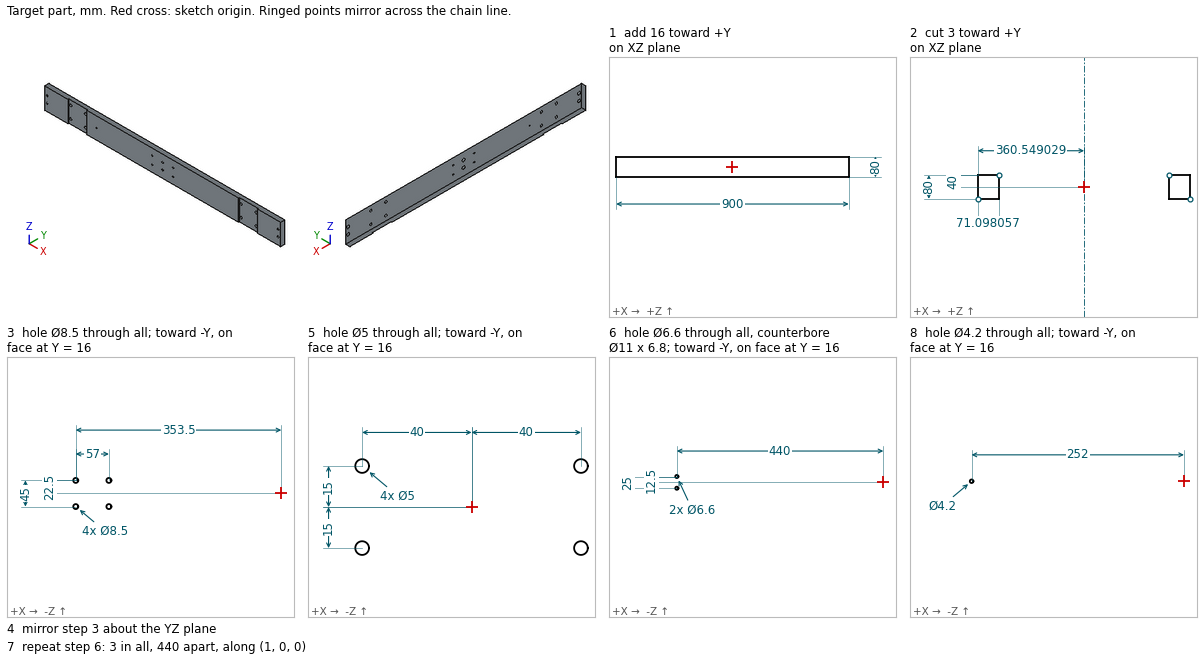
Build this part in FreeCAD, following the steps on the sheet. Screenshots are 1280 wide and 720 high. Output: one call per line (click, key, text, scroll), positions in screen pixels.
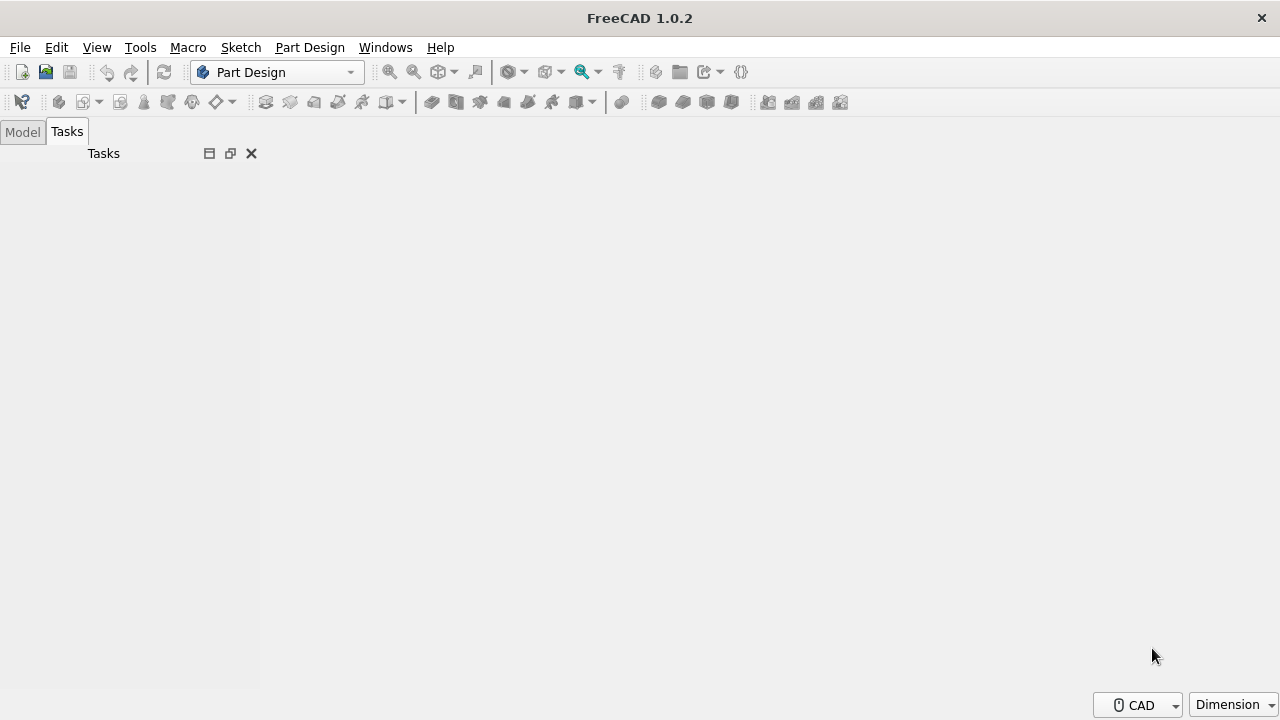
click(22, 72)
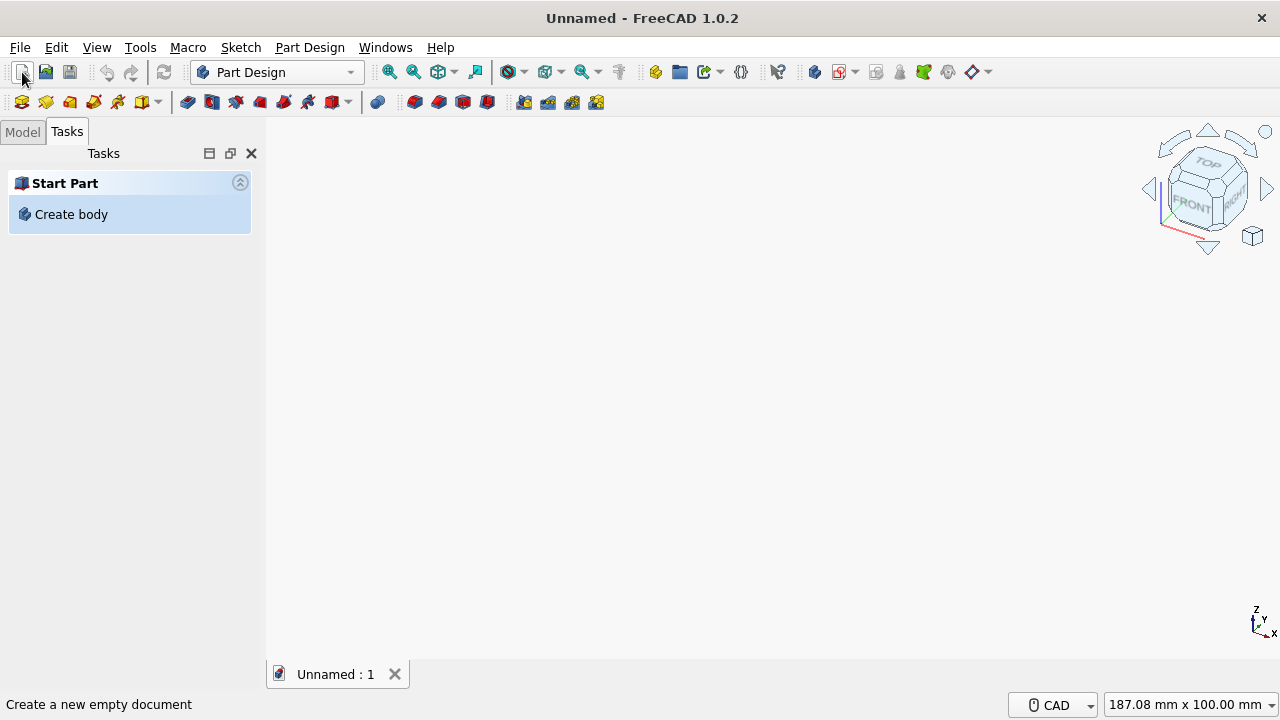
click(840, 72)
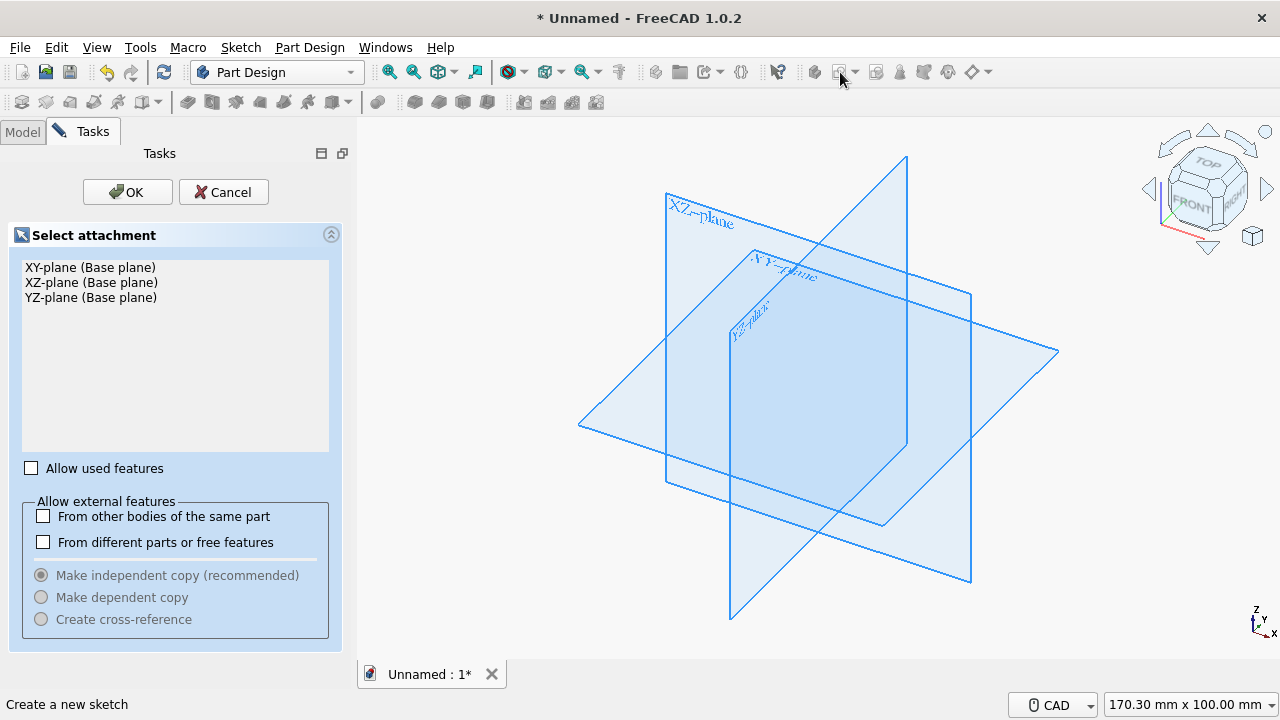
click(82, 282)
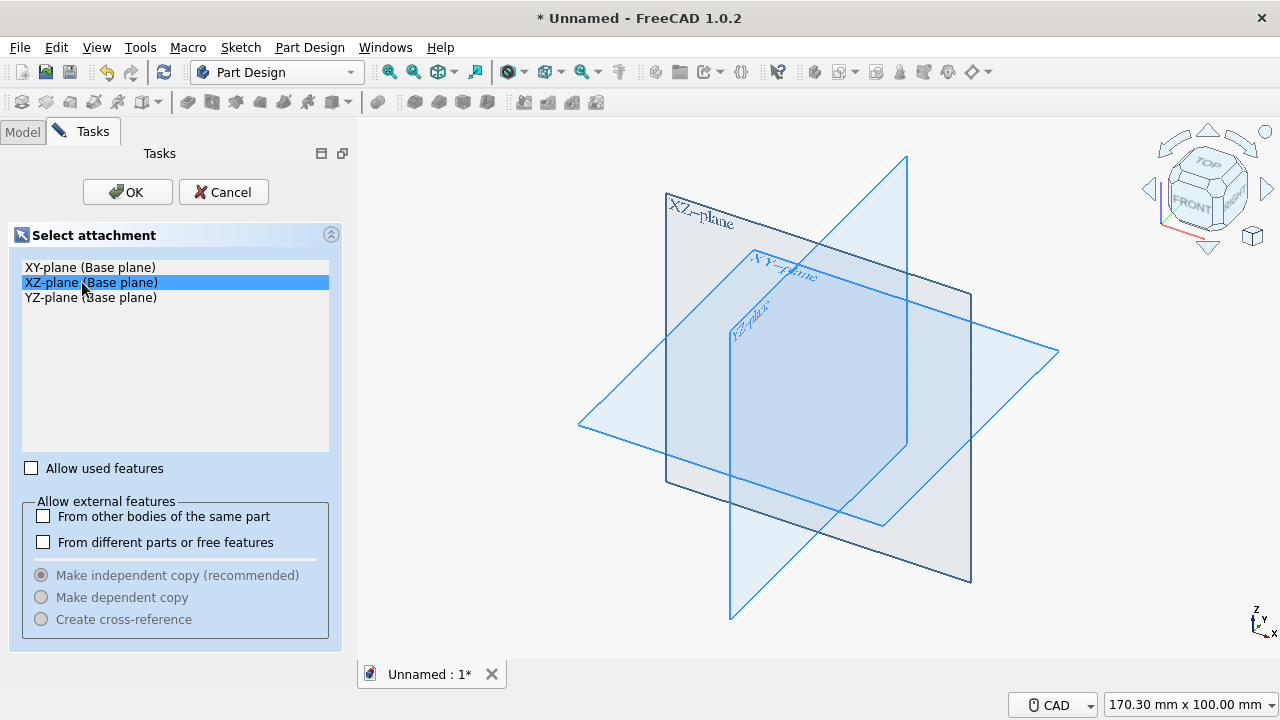
click(128, 192)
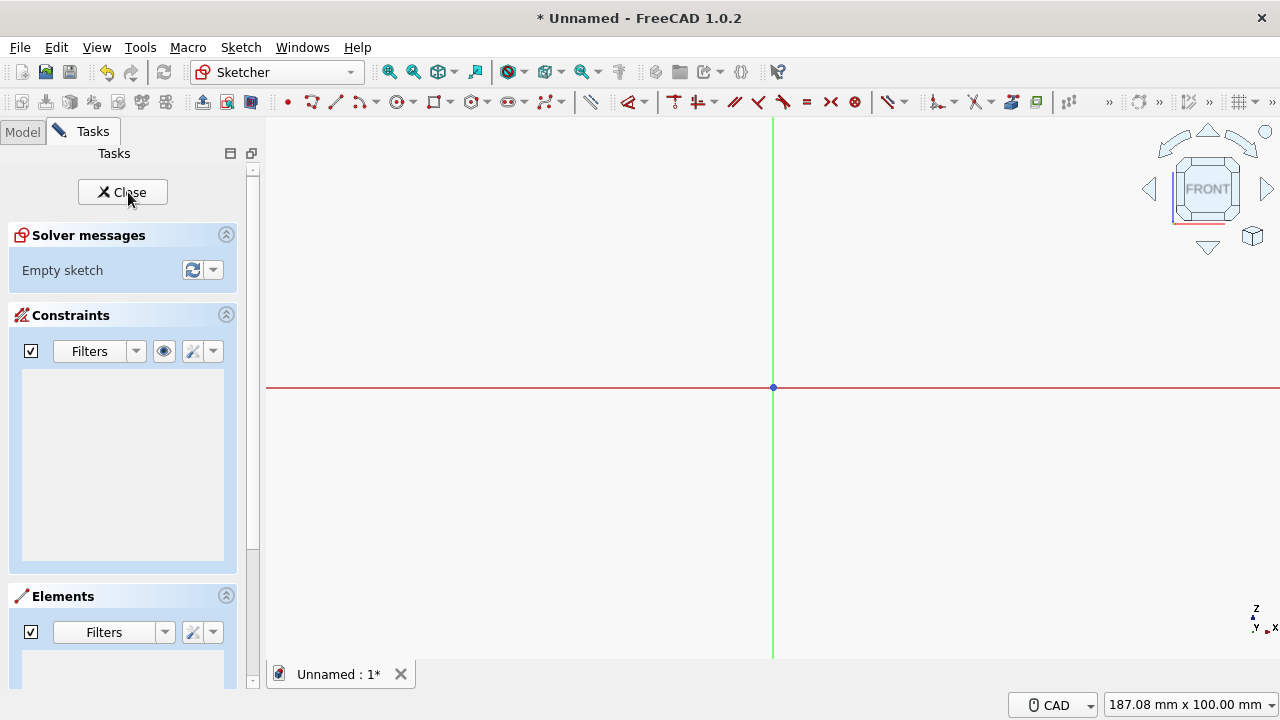
scroll(696, 388, down, 11)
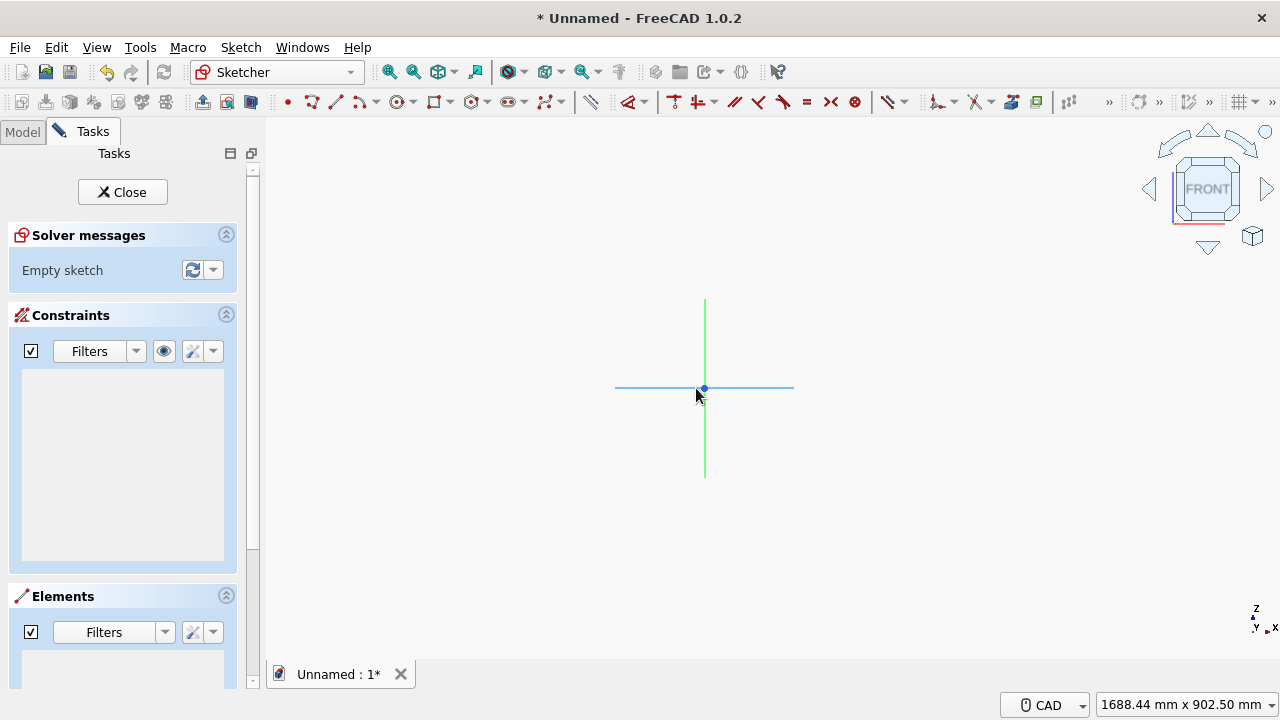
key(g)
key(v)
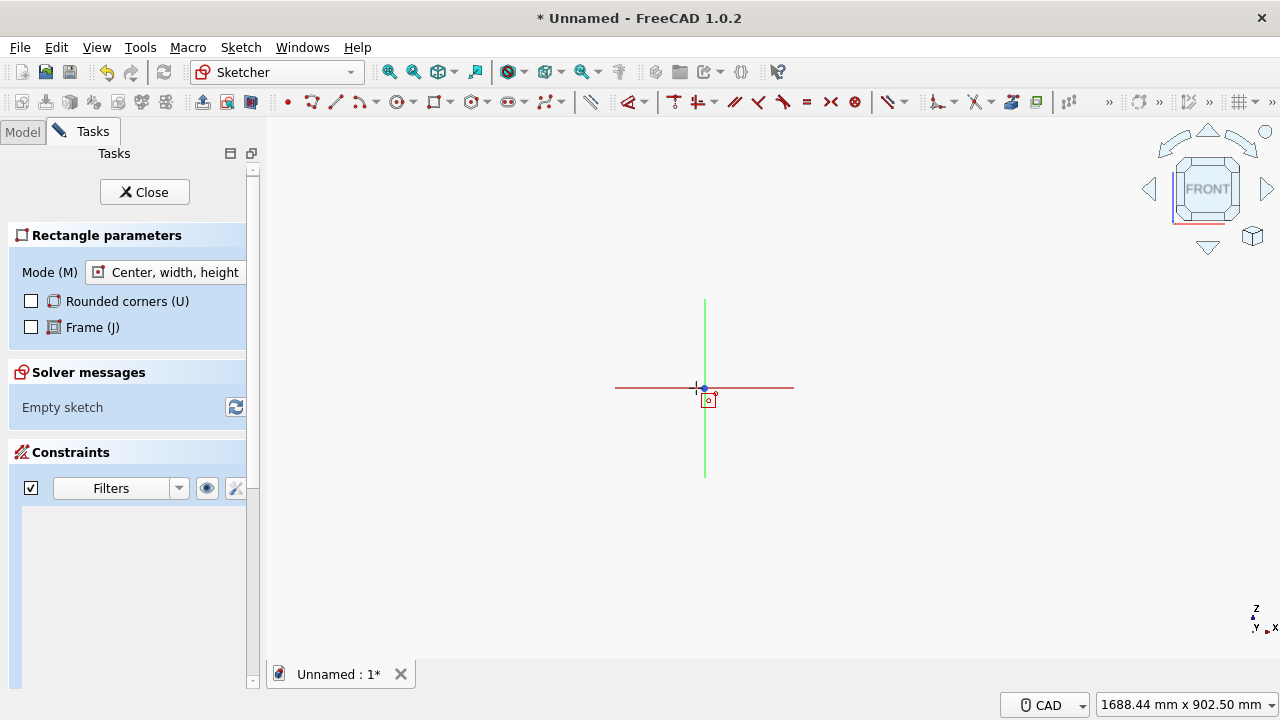
click(705, 388)
click(975, 364)
key(Escape)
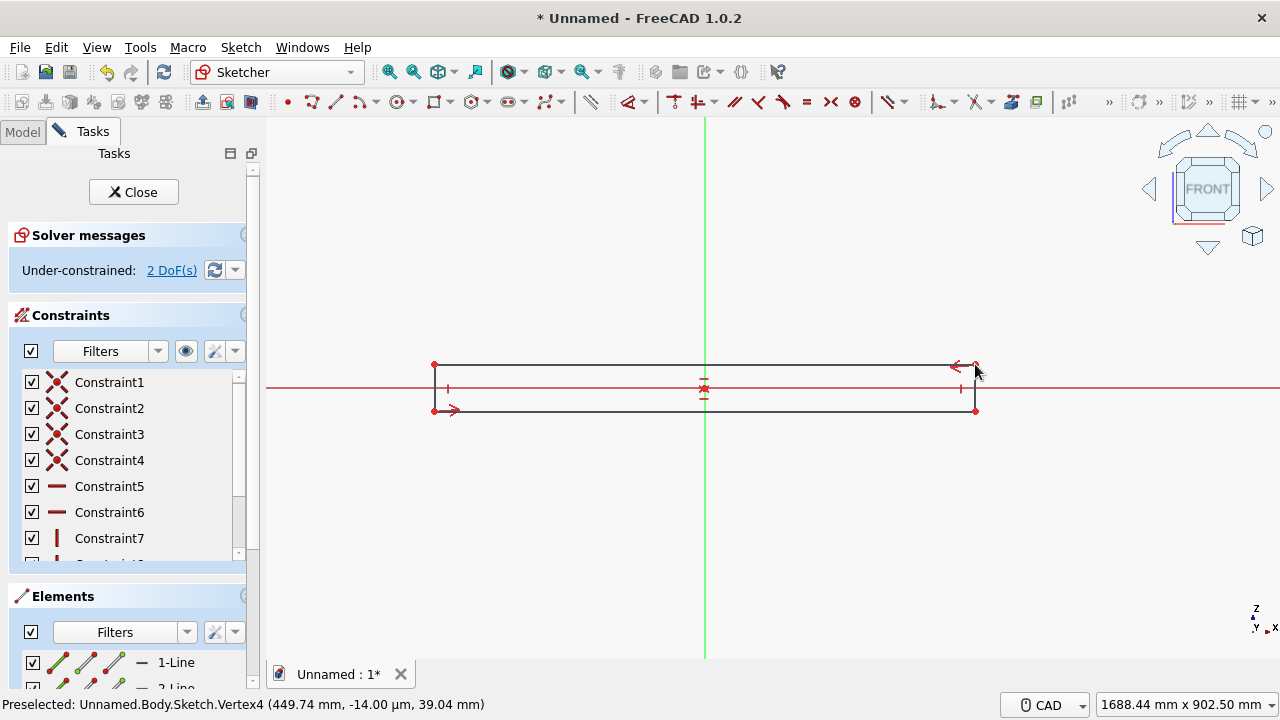
click(628, 102)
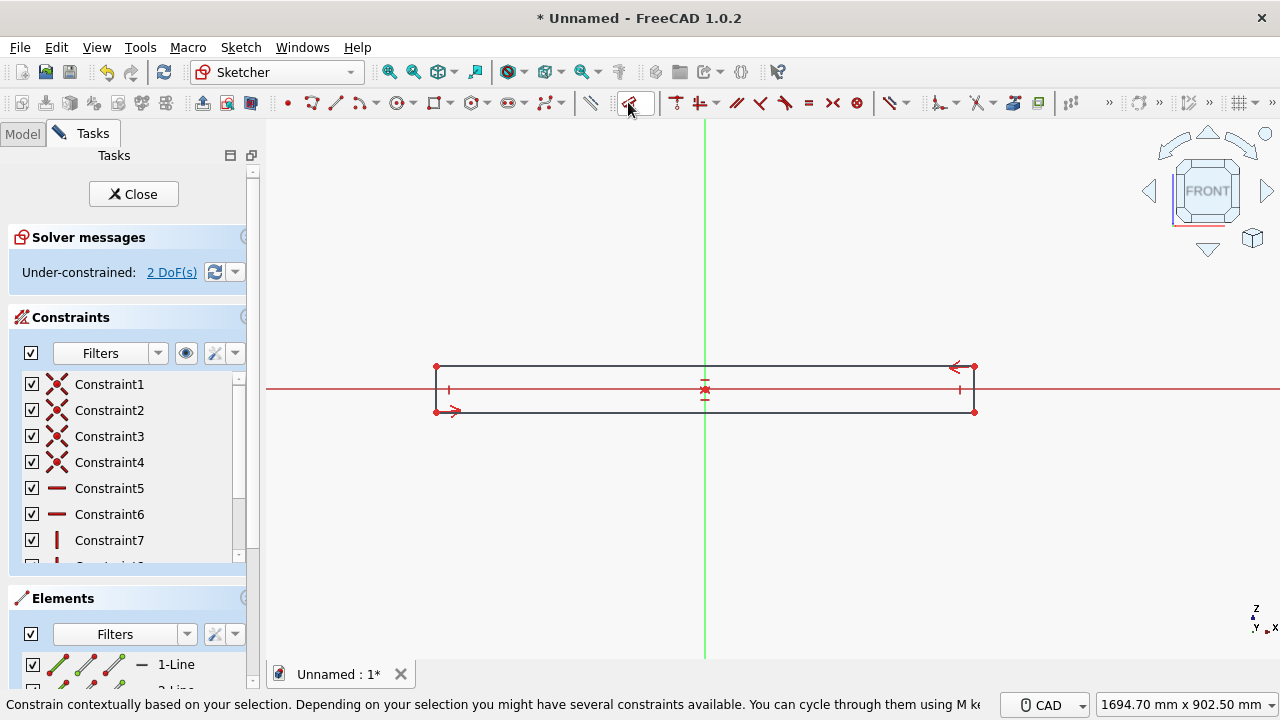
scroll(974, 399, up, 2)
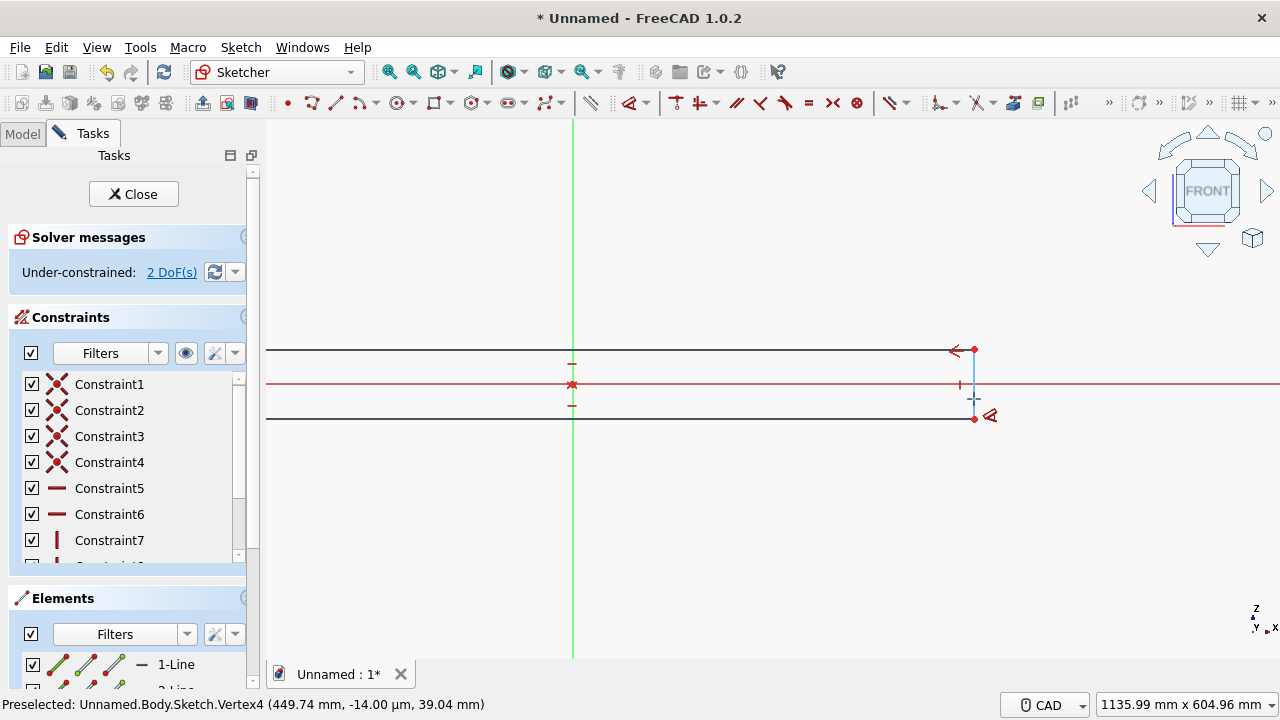
click(974, 398)
click(1008, 368)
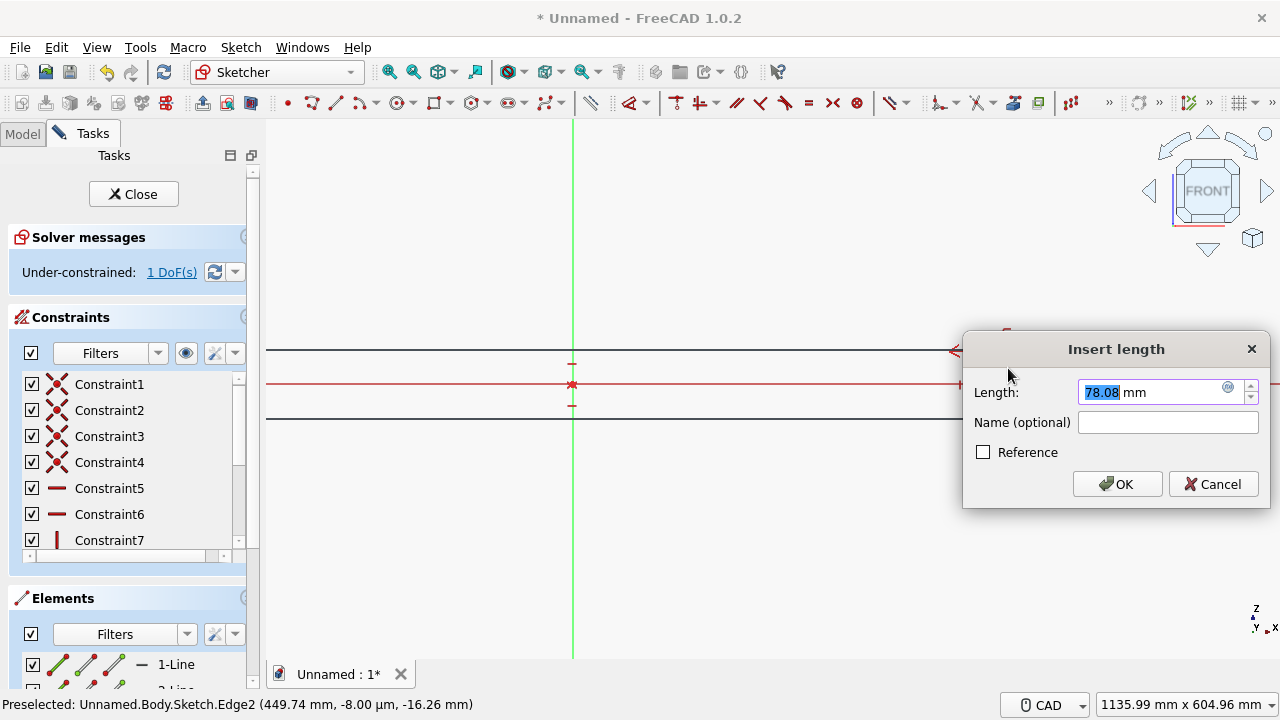
text(80)
key(Return)